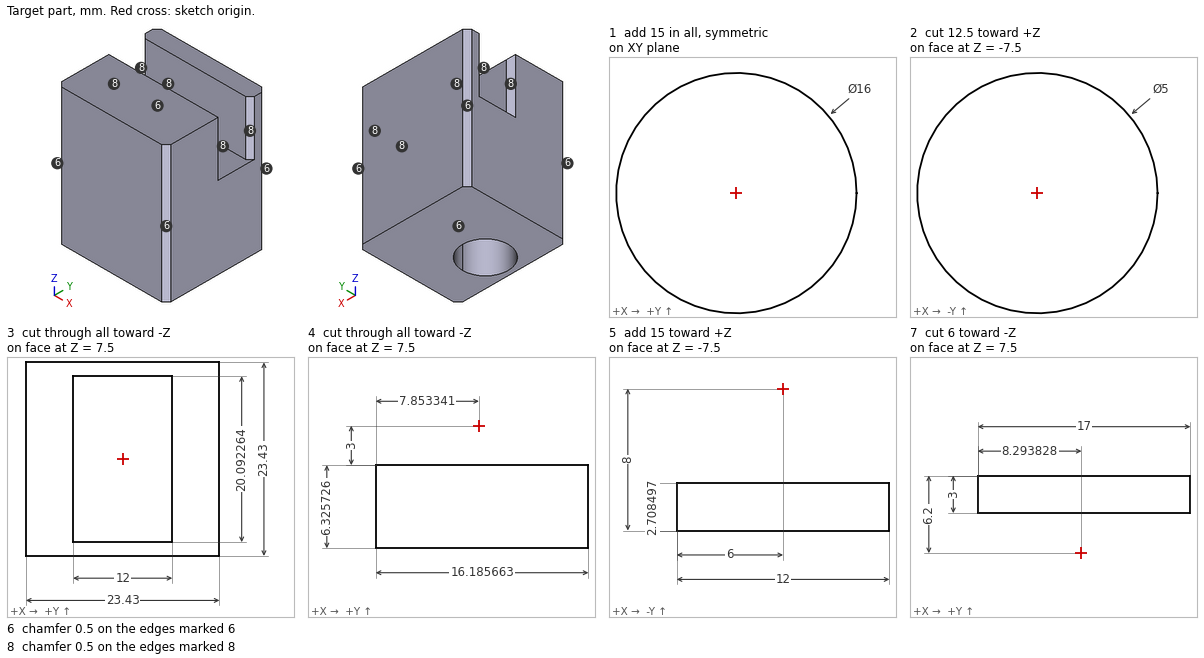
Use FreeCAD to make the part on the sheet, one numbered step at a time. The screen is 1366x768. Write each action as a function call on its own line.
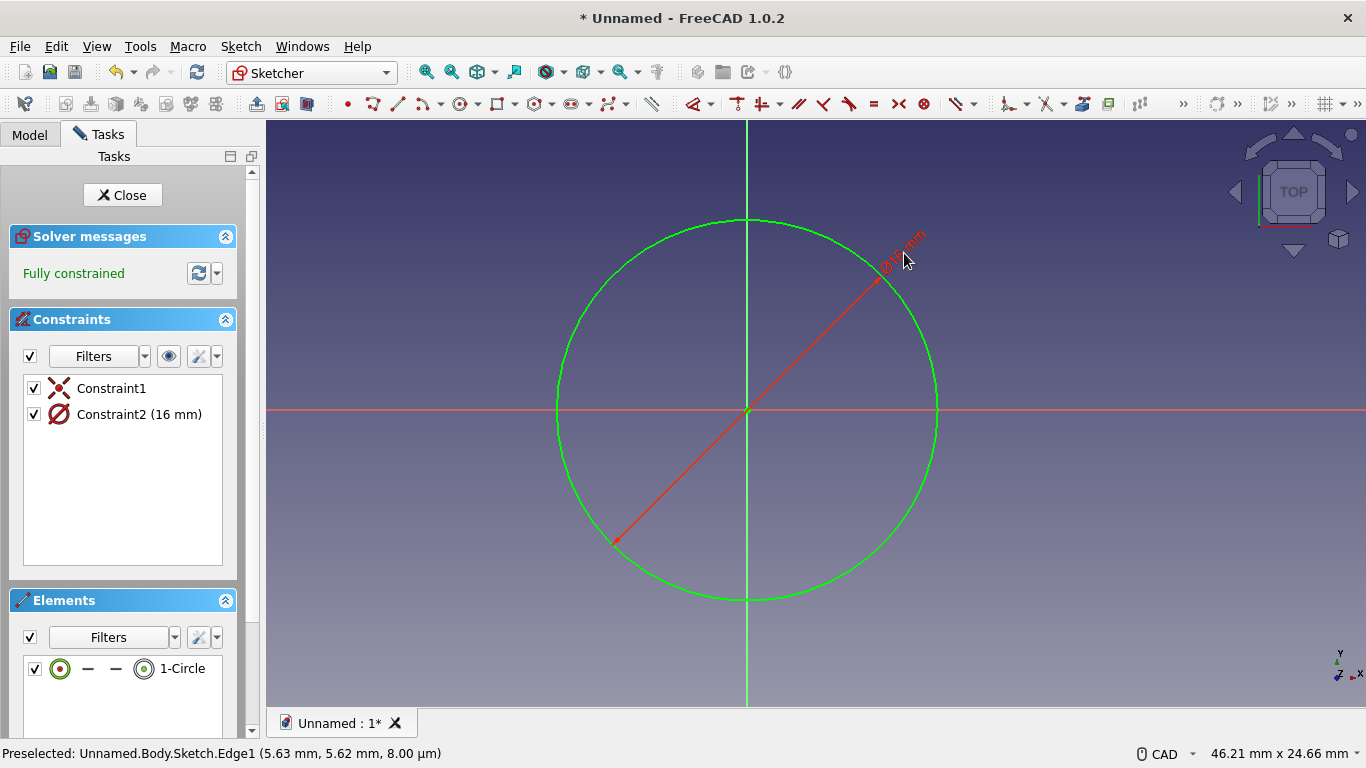
click(123, 195)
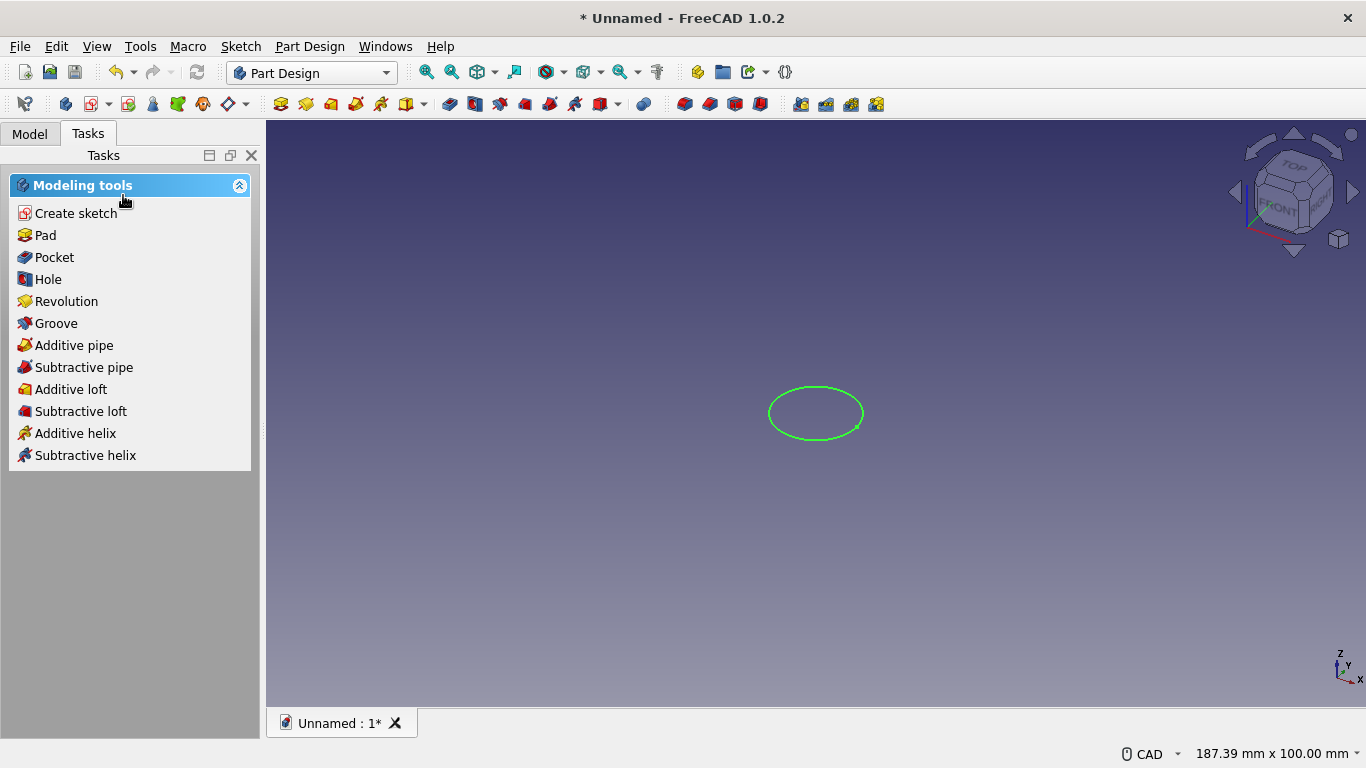
click(281, 104)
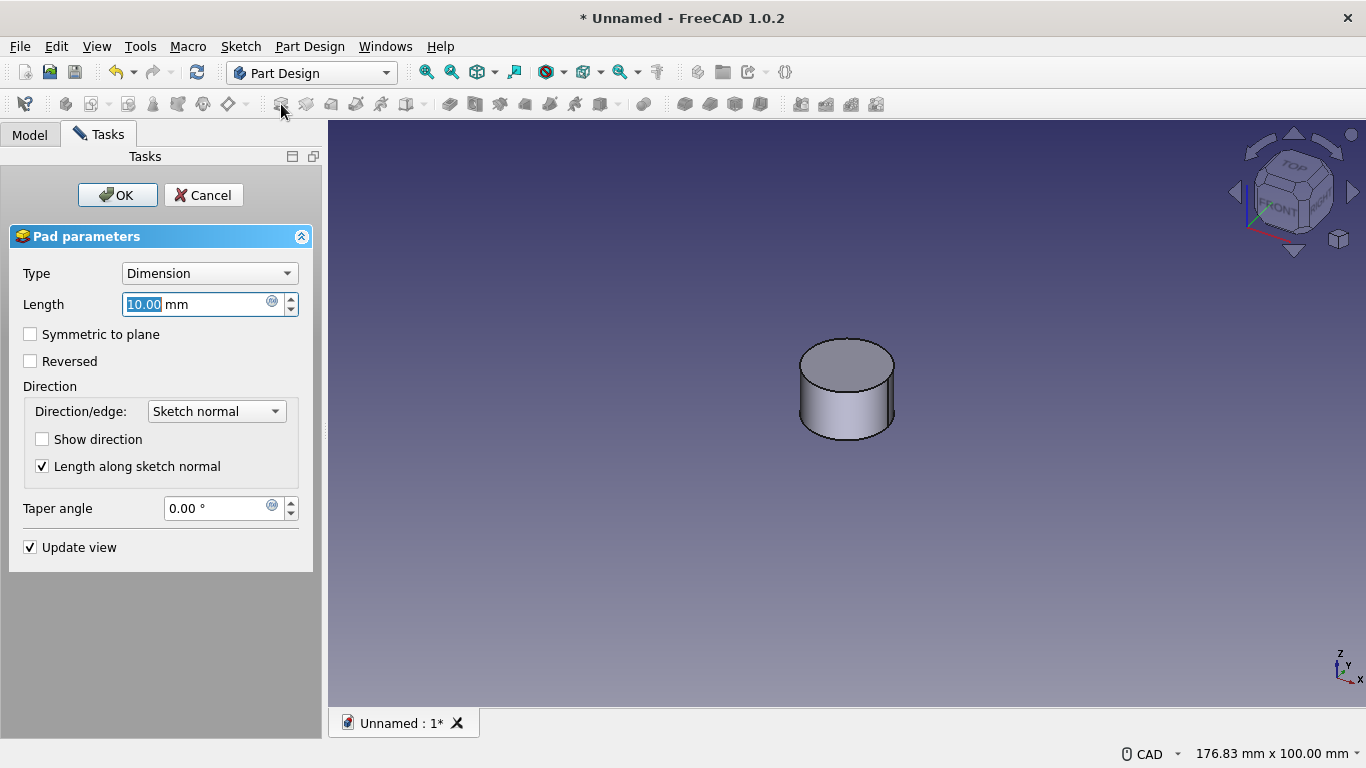
text(15)
key(Tab)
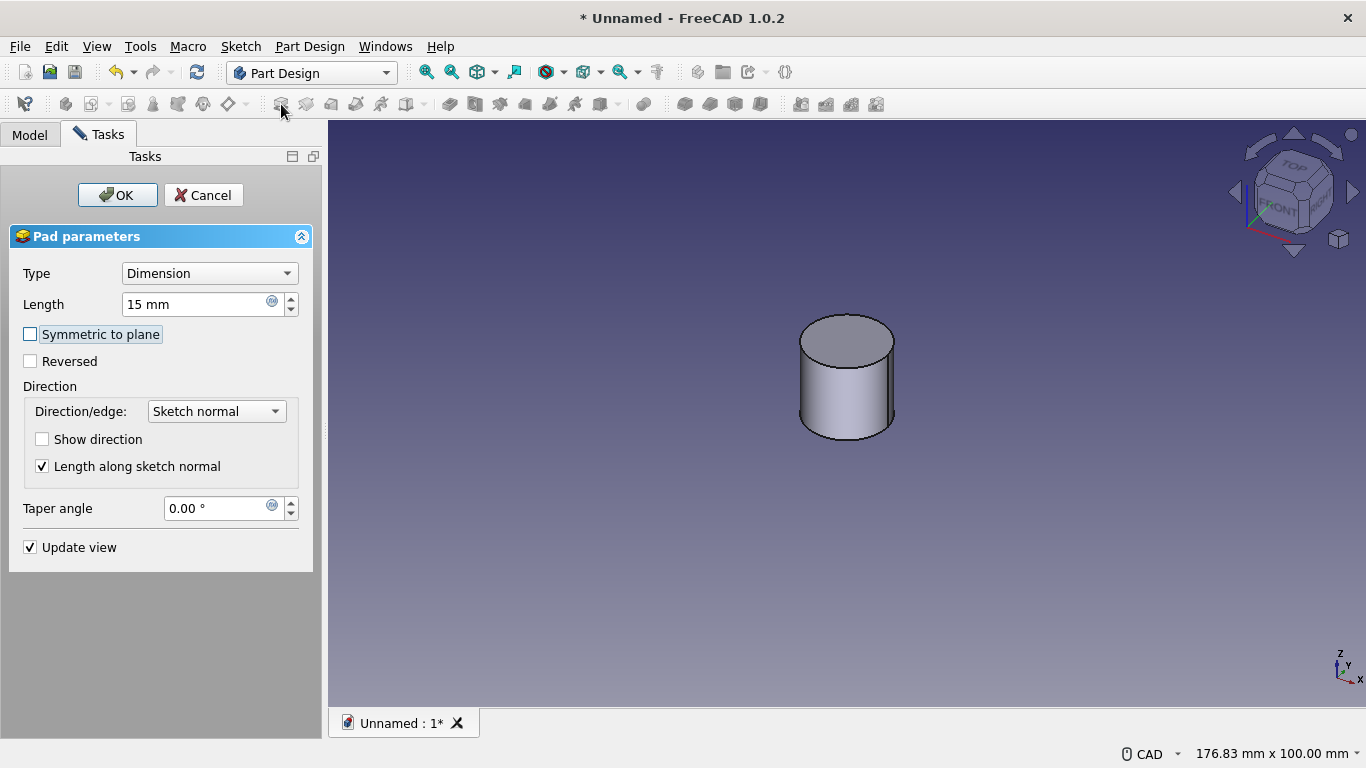
click(31, 334)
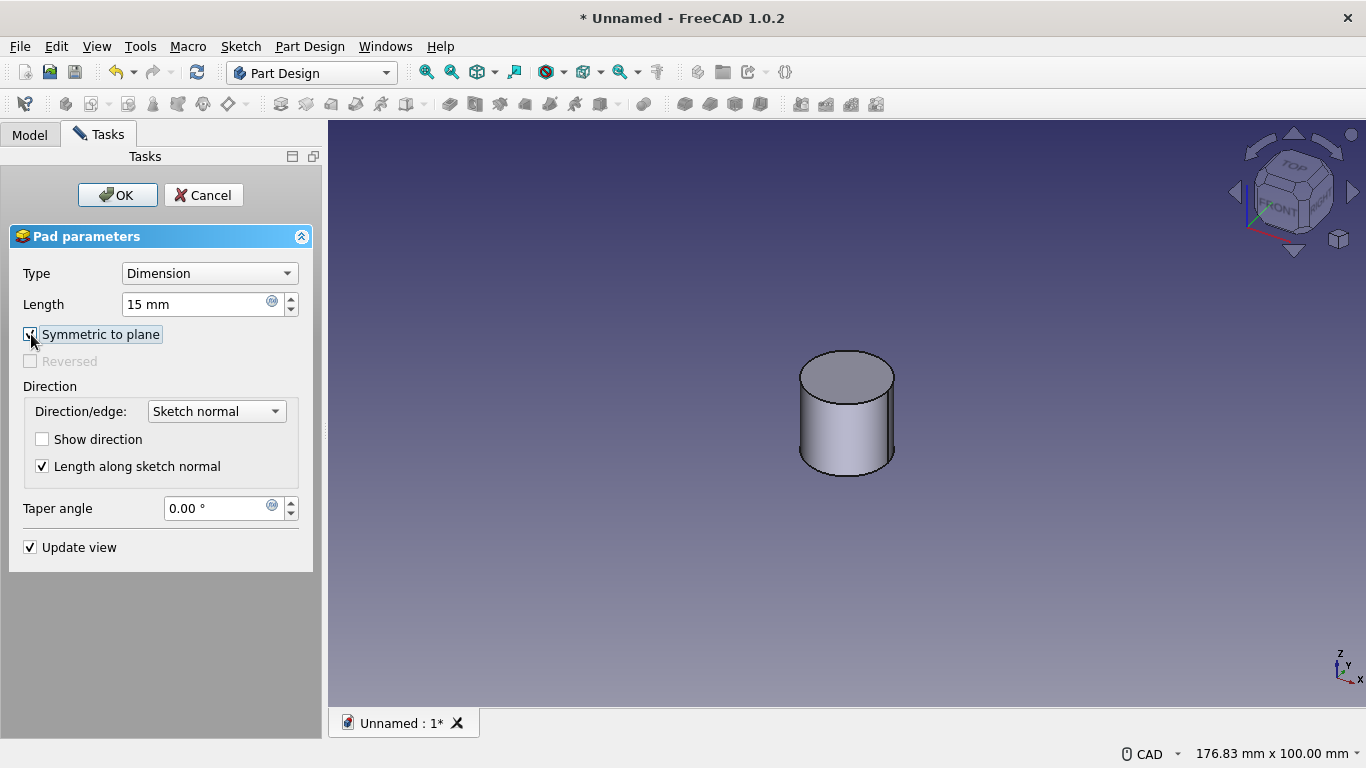
click(118, 195)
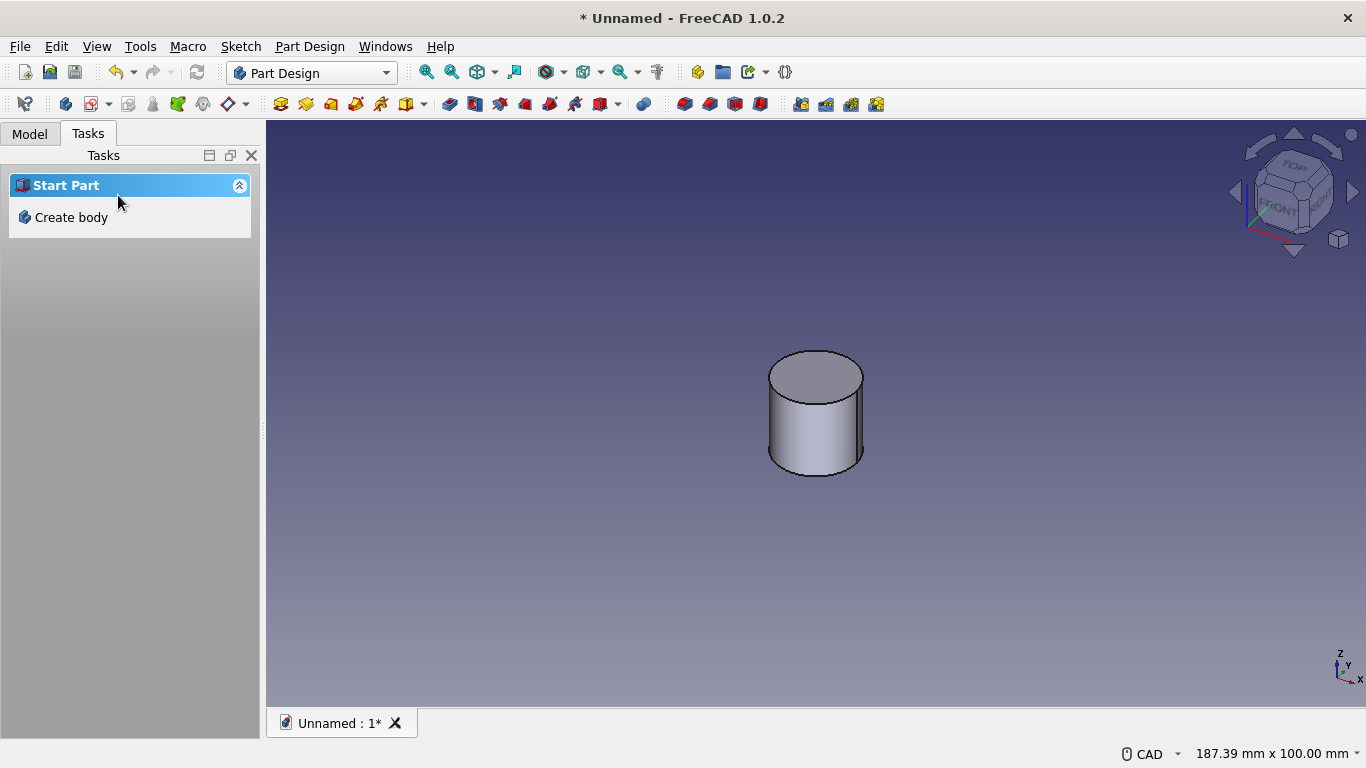
click(427, 72)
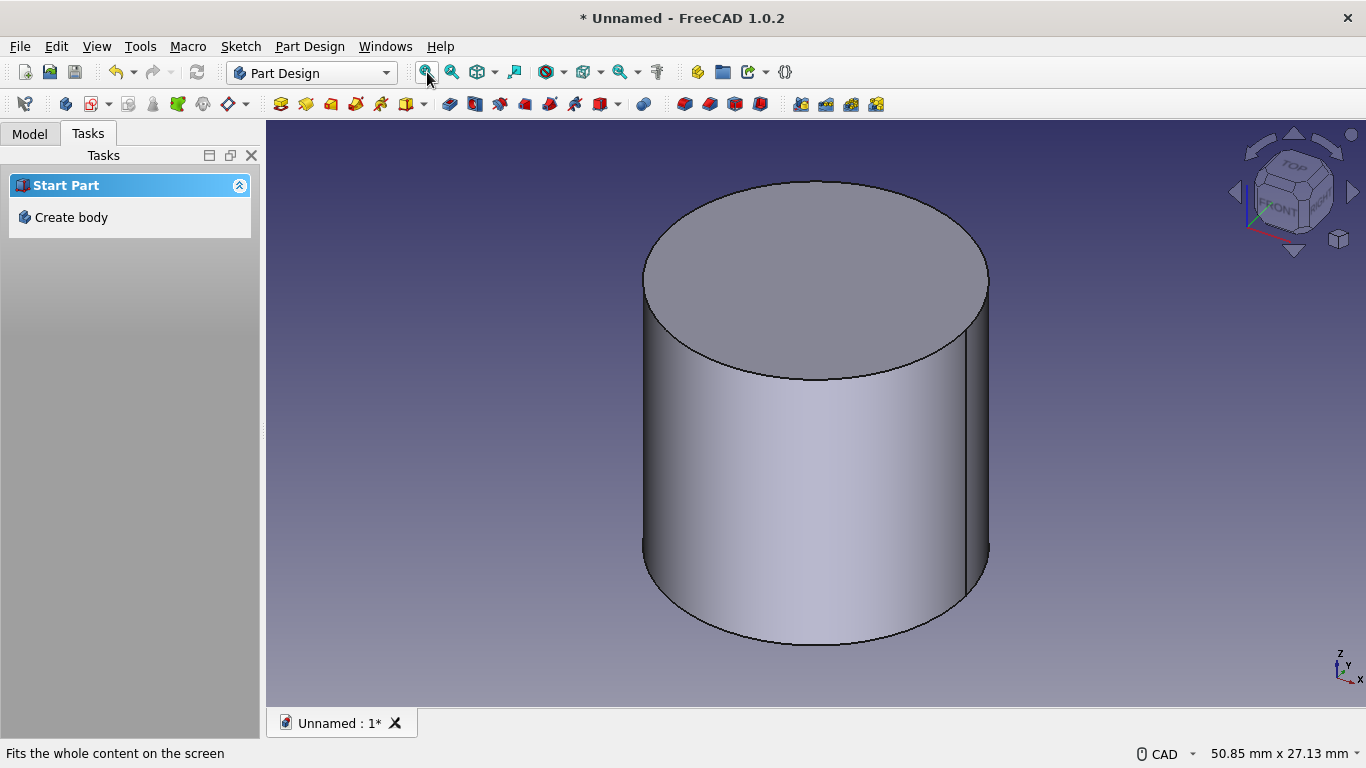
key(5)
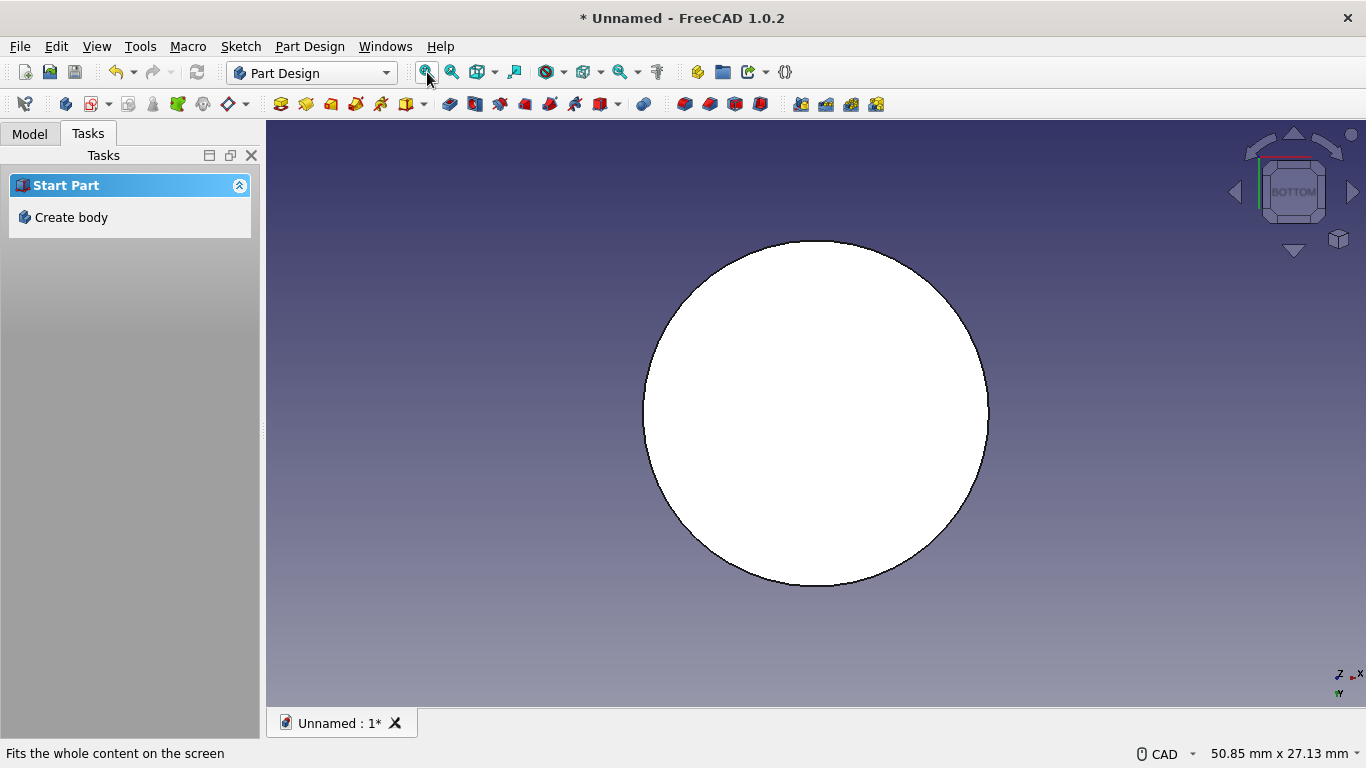
click(816, 412)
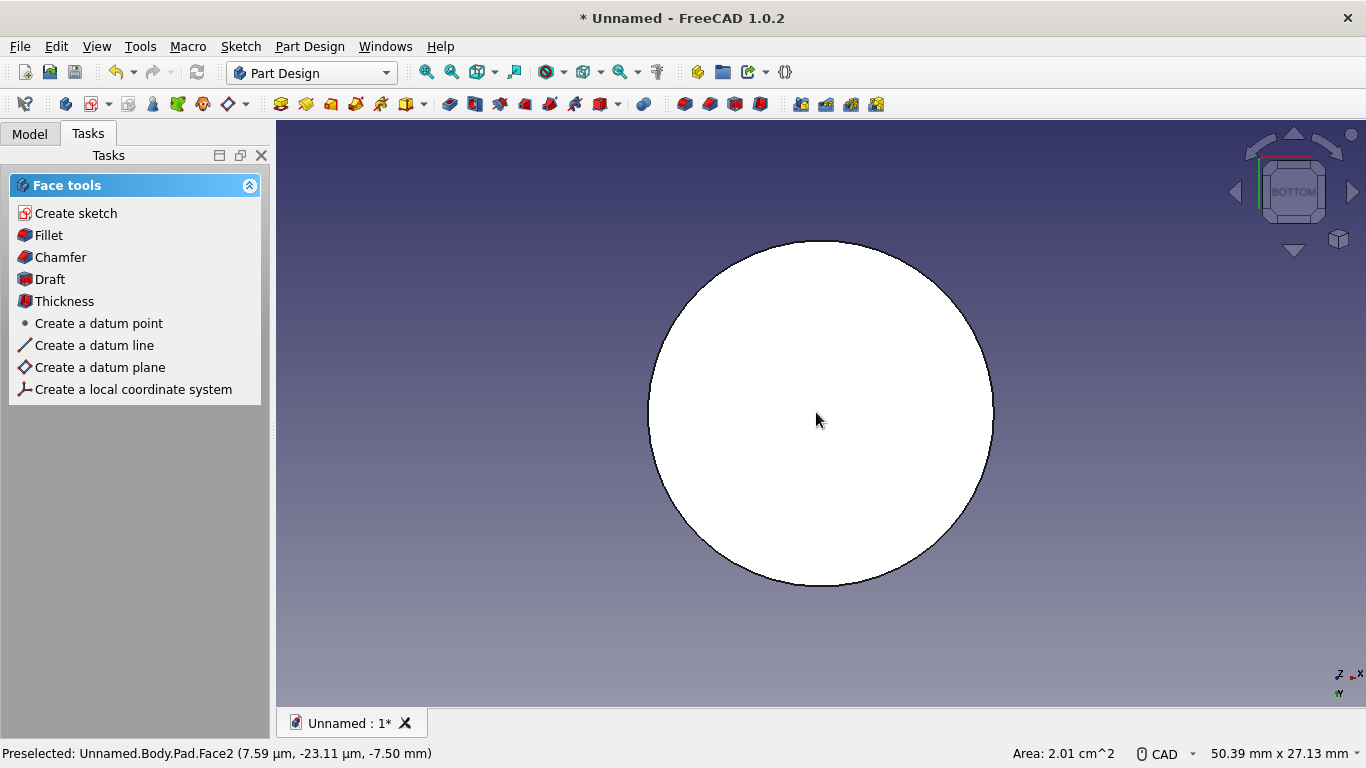
click(90, 104)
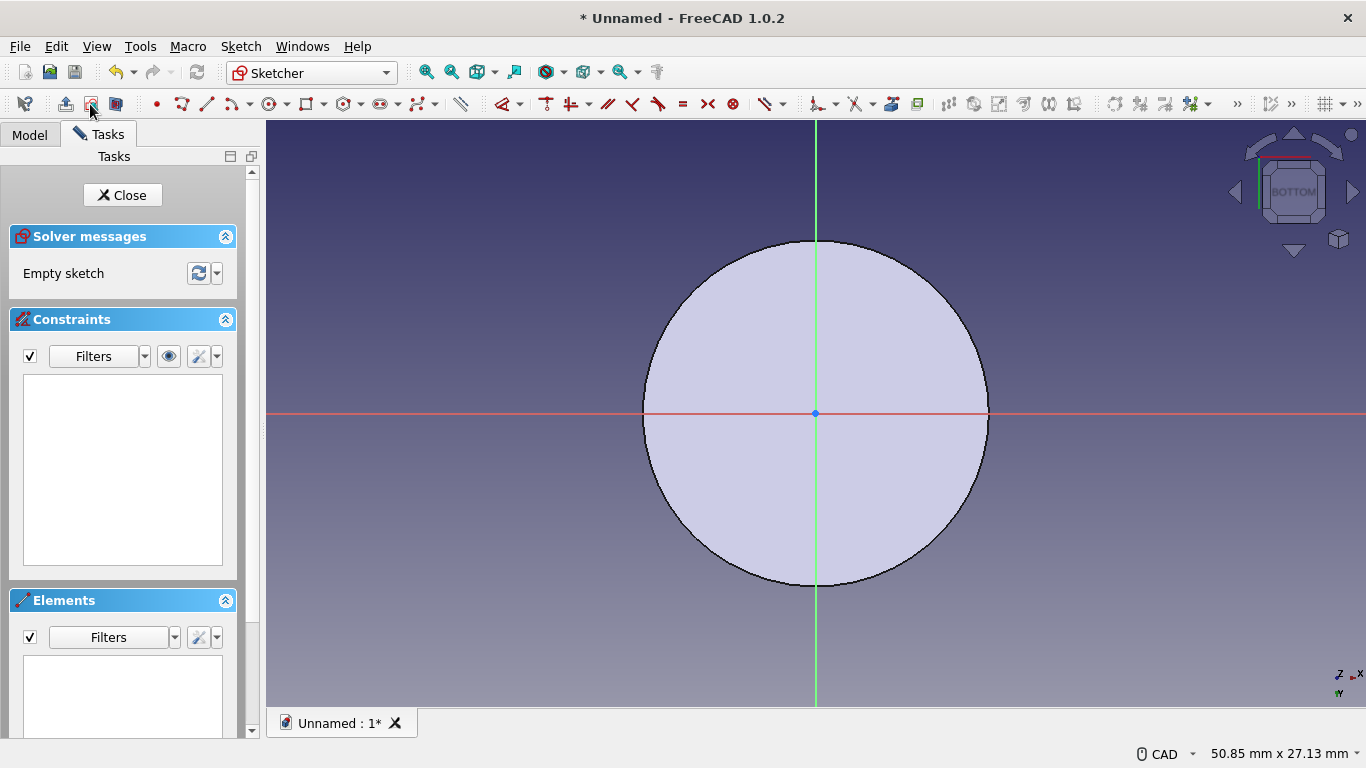
scroll(845, 414, up, 6)